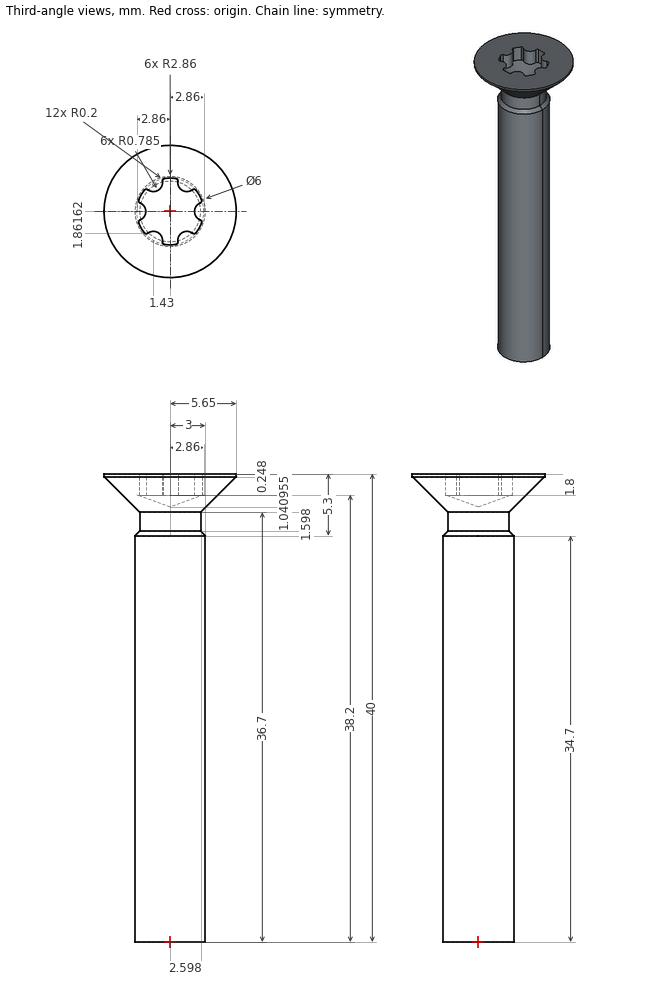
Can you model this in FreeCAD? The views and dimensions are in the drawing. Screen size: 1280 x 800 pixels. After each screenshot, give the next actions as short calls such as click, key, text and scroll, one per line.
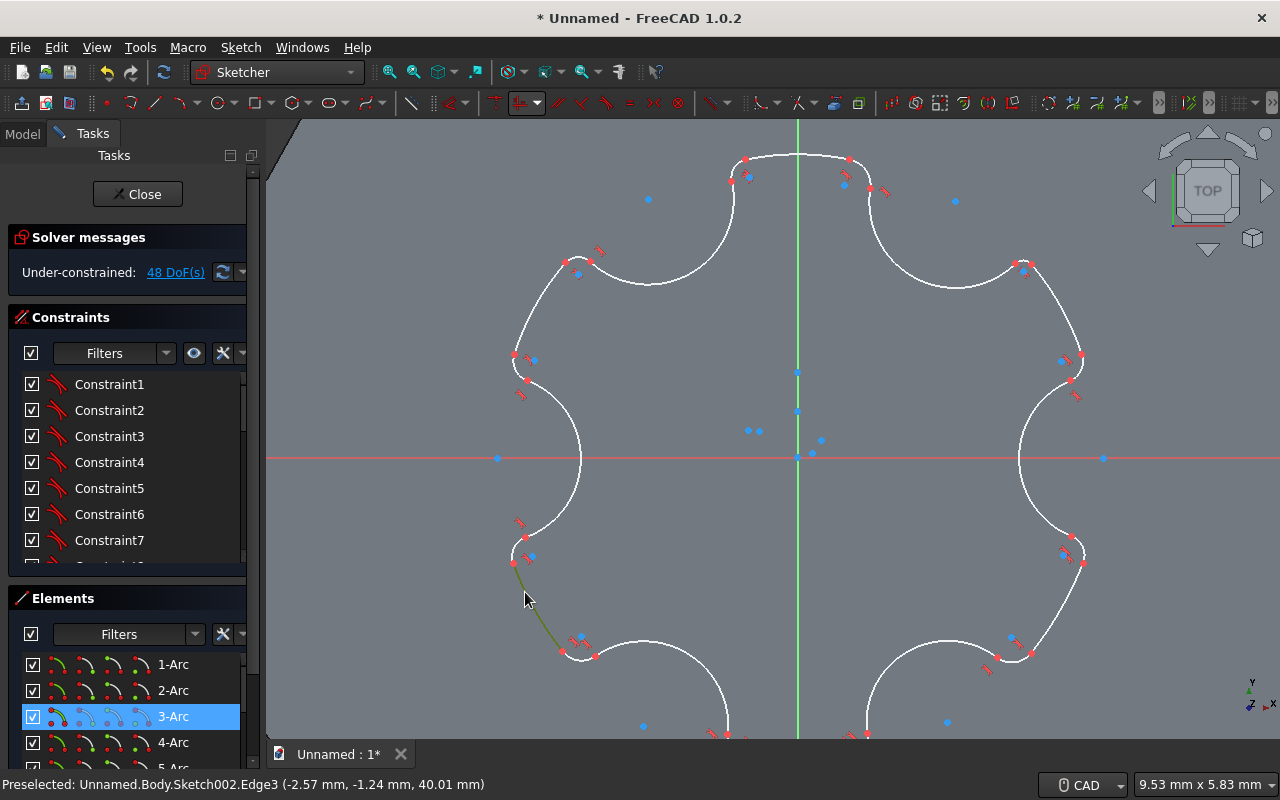
scroll(515, 371, down, 2)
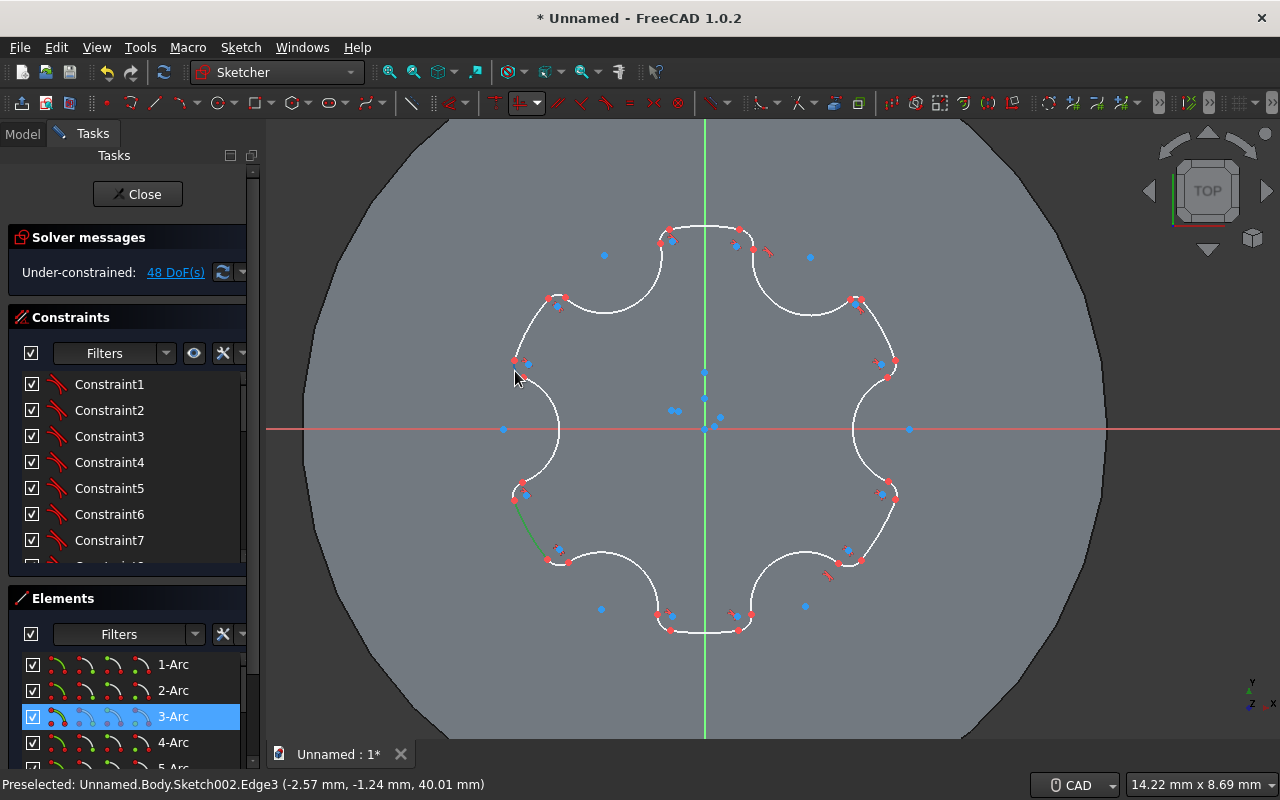
click(691, 633)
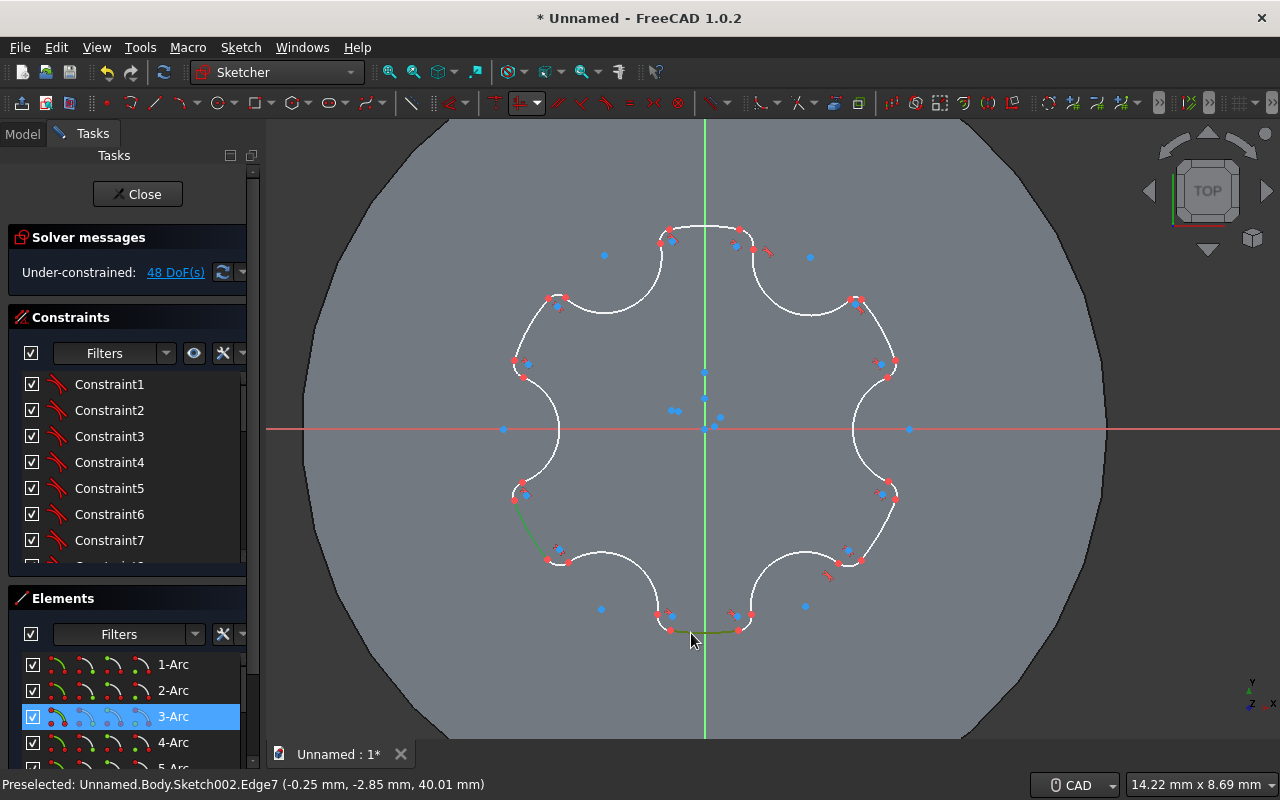
click(496, 104)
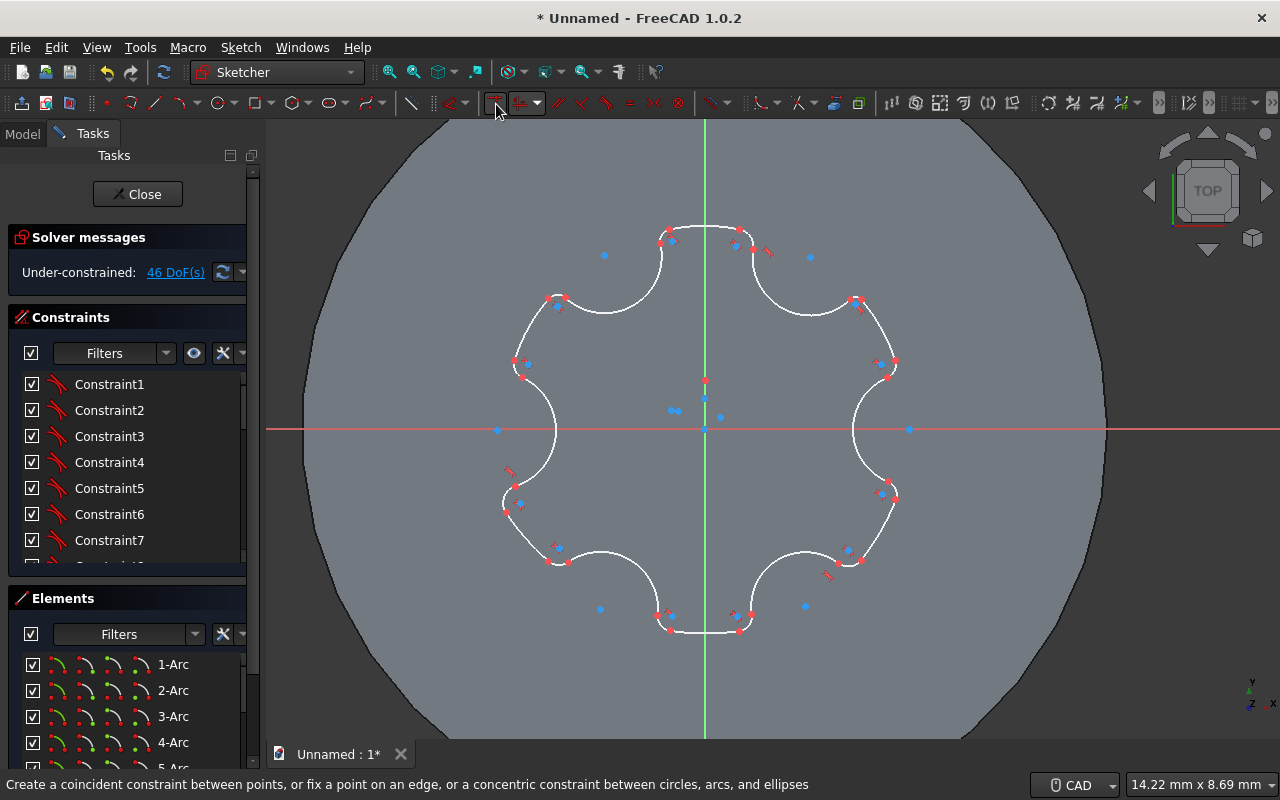
click(517, 528)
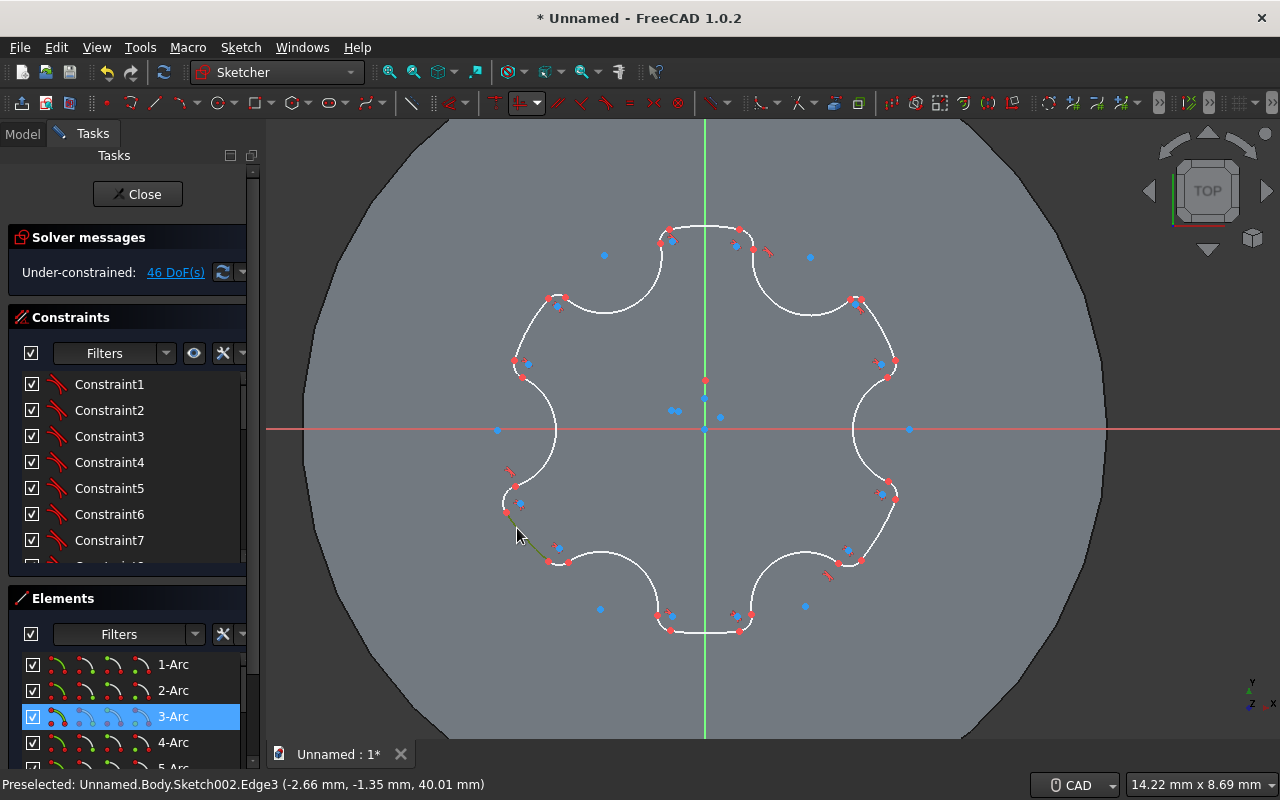
click(873, 543)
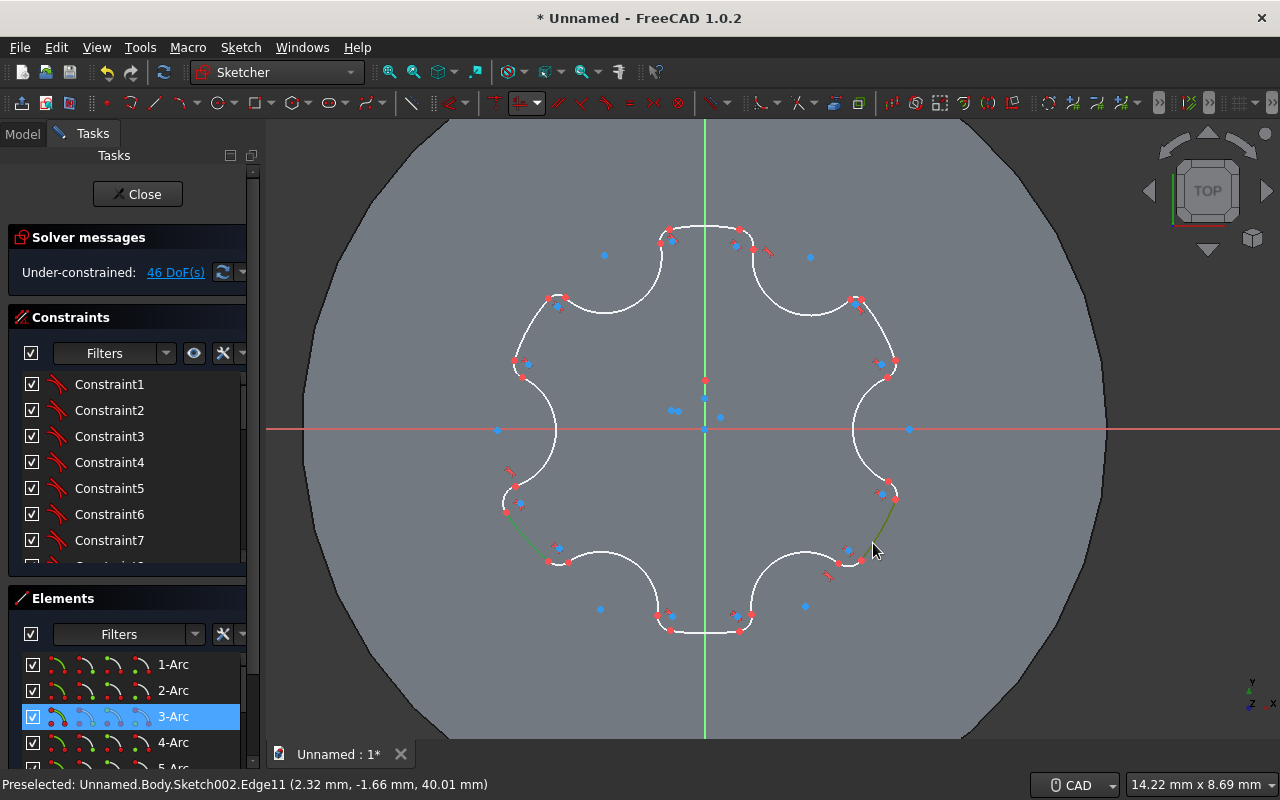
click(496, 104)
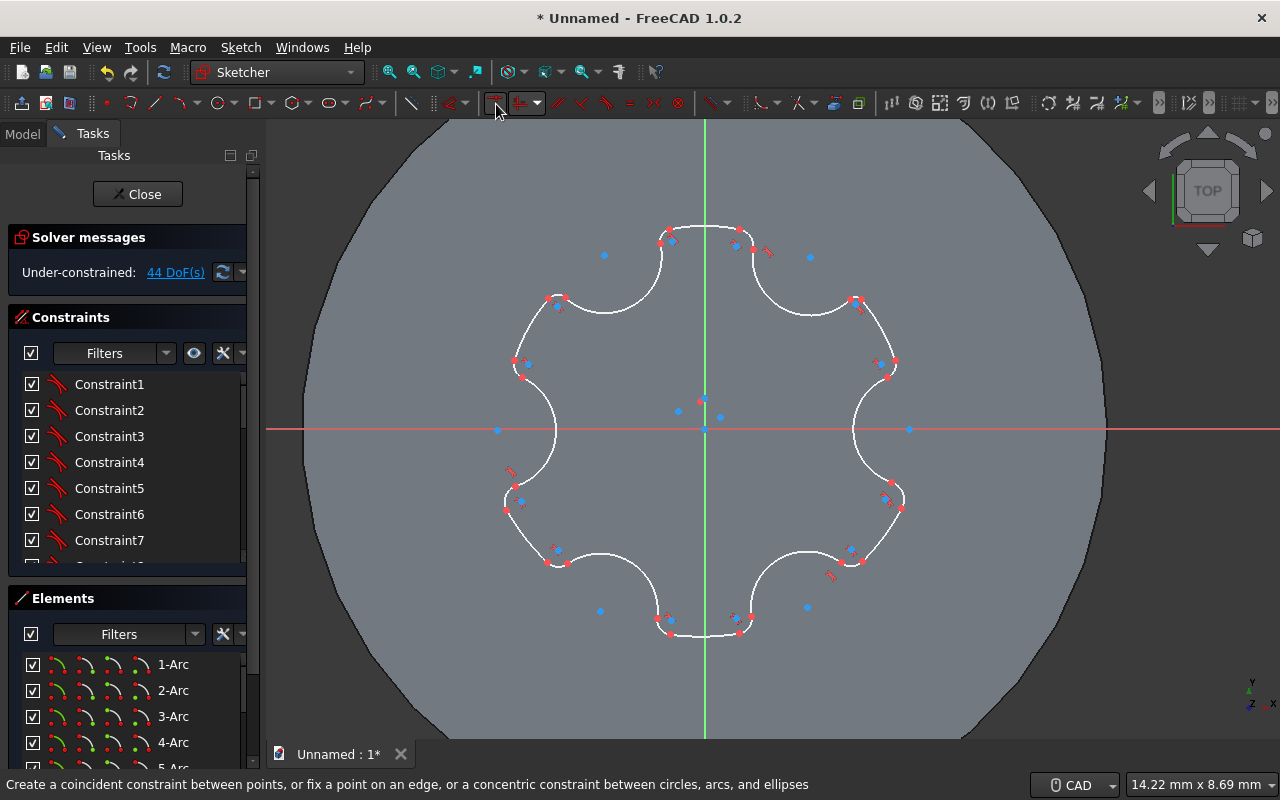
click(517, 527)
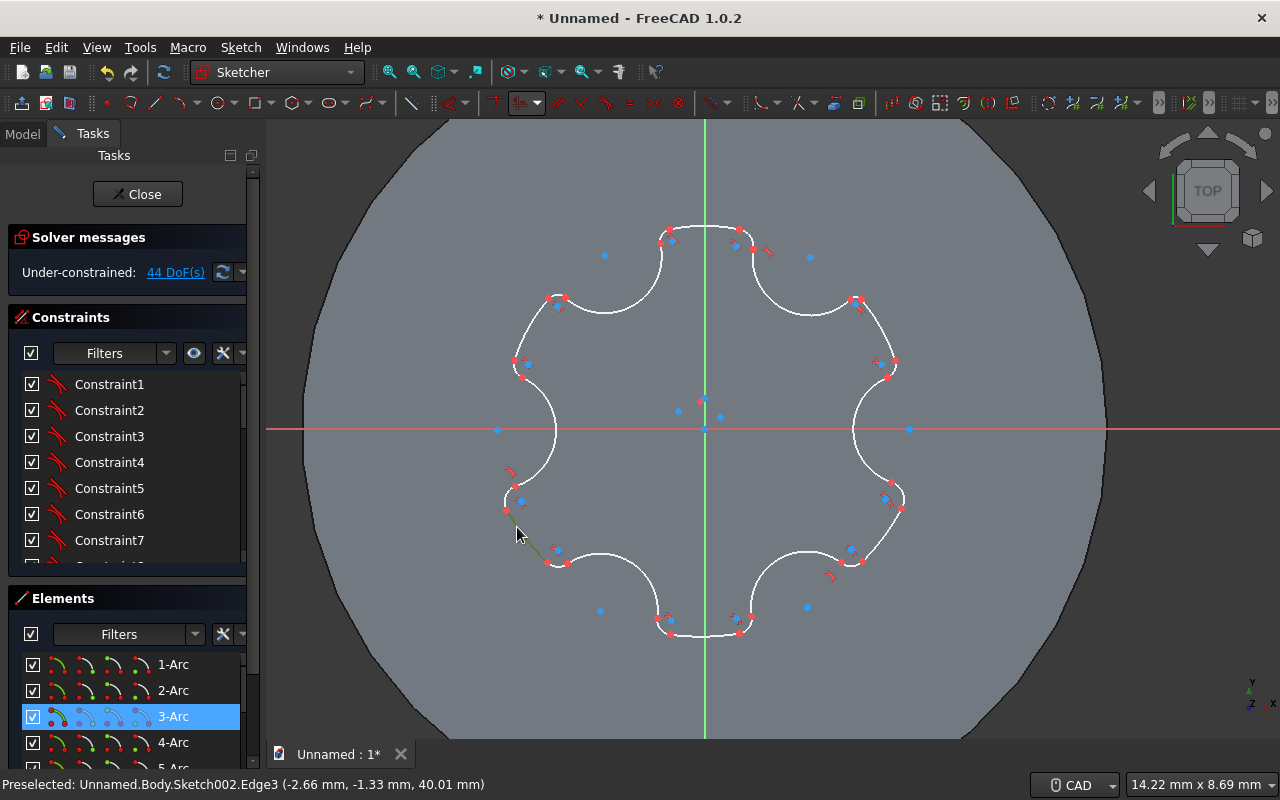
click(887, 341)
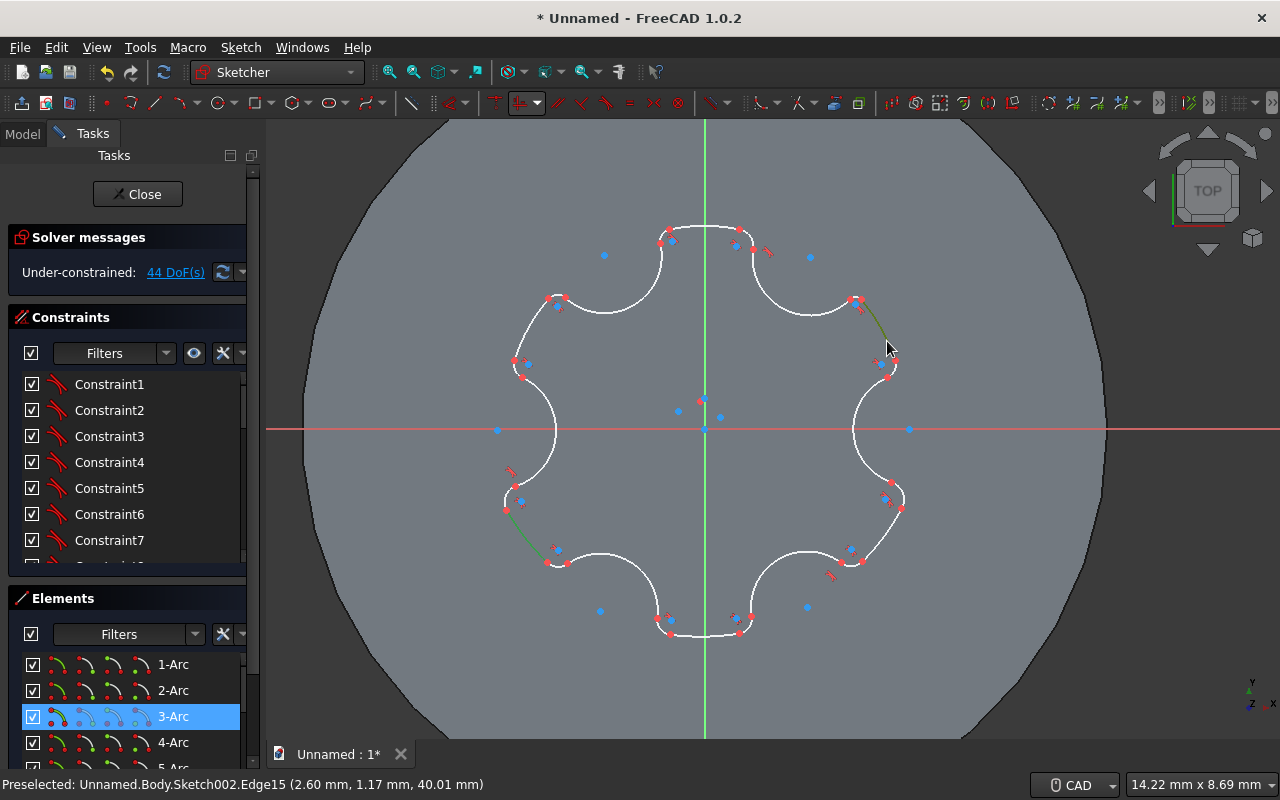
key(c)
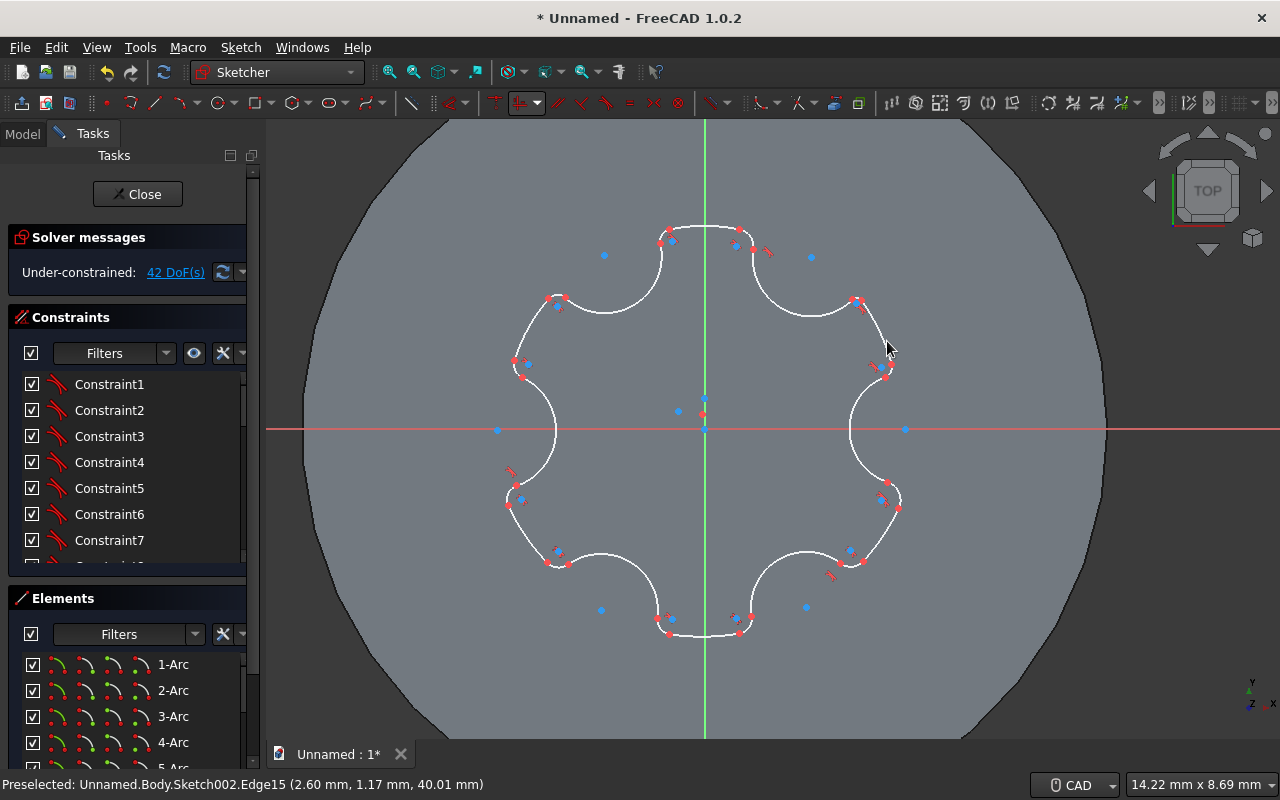
click(518, 524)